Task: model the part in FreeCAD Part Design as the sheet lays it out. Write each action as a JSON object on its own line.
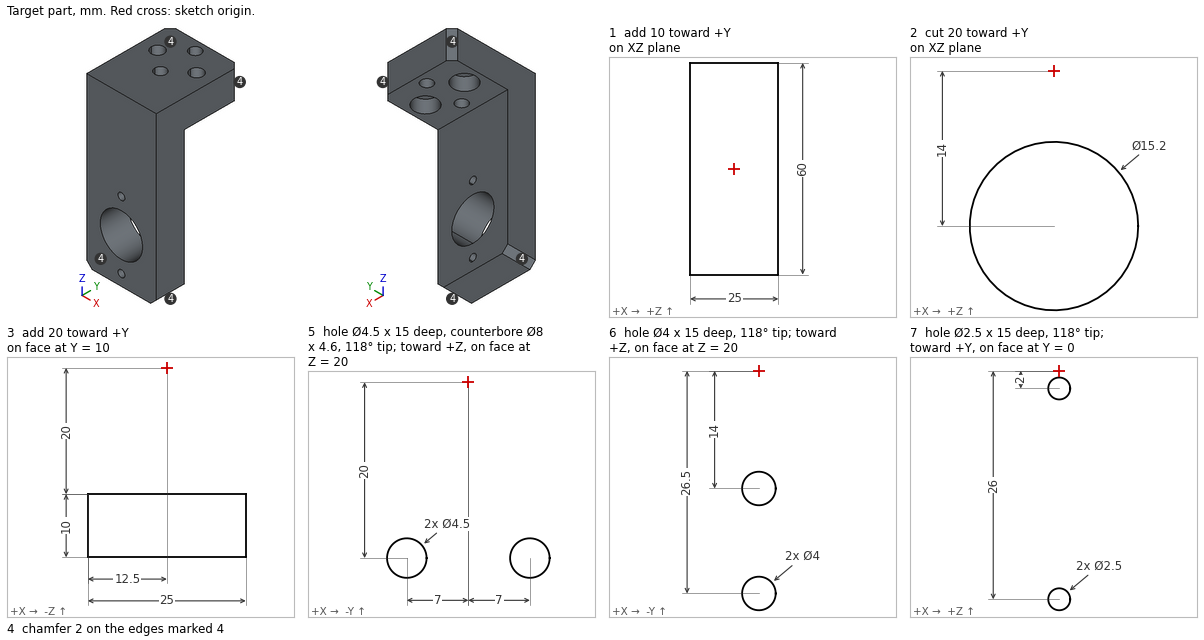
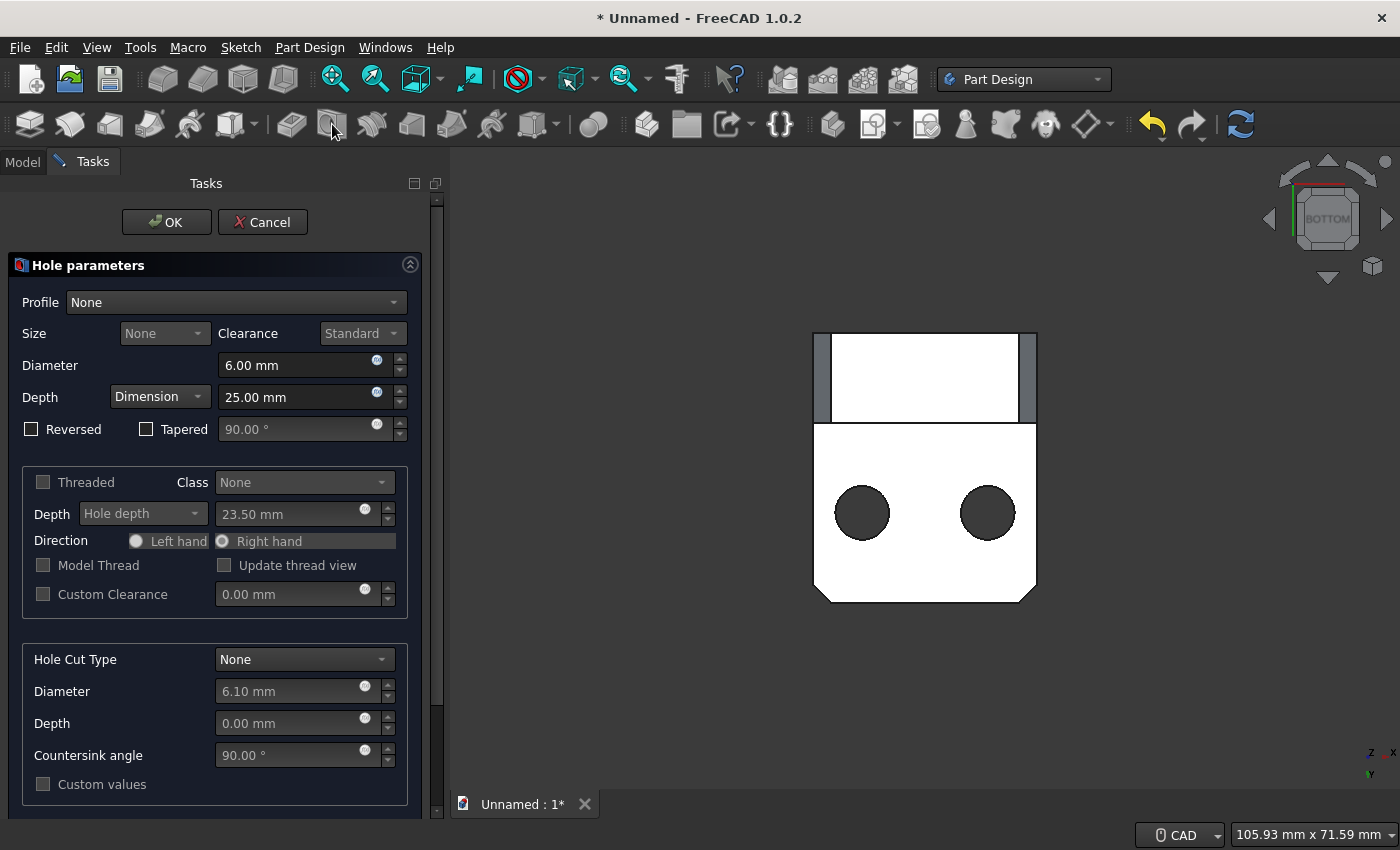
{"action": "triple_click", "coordinate": [305, 365]}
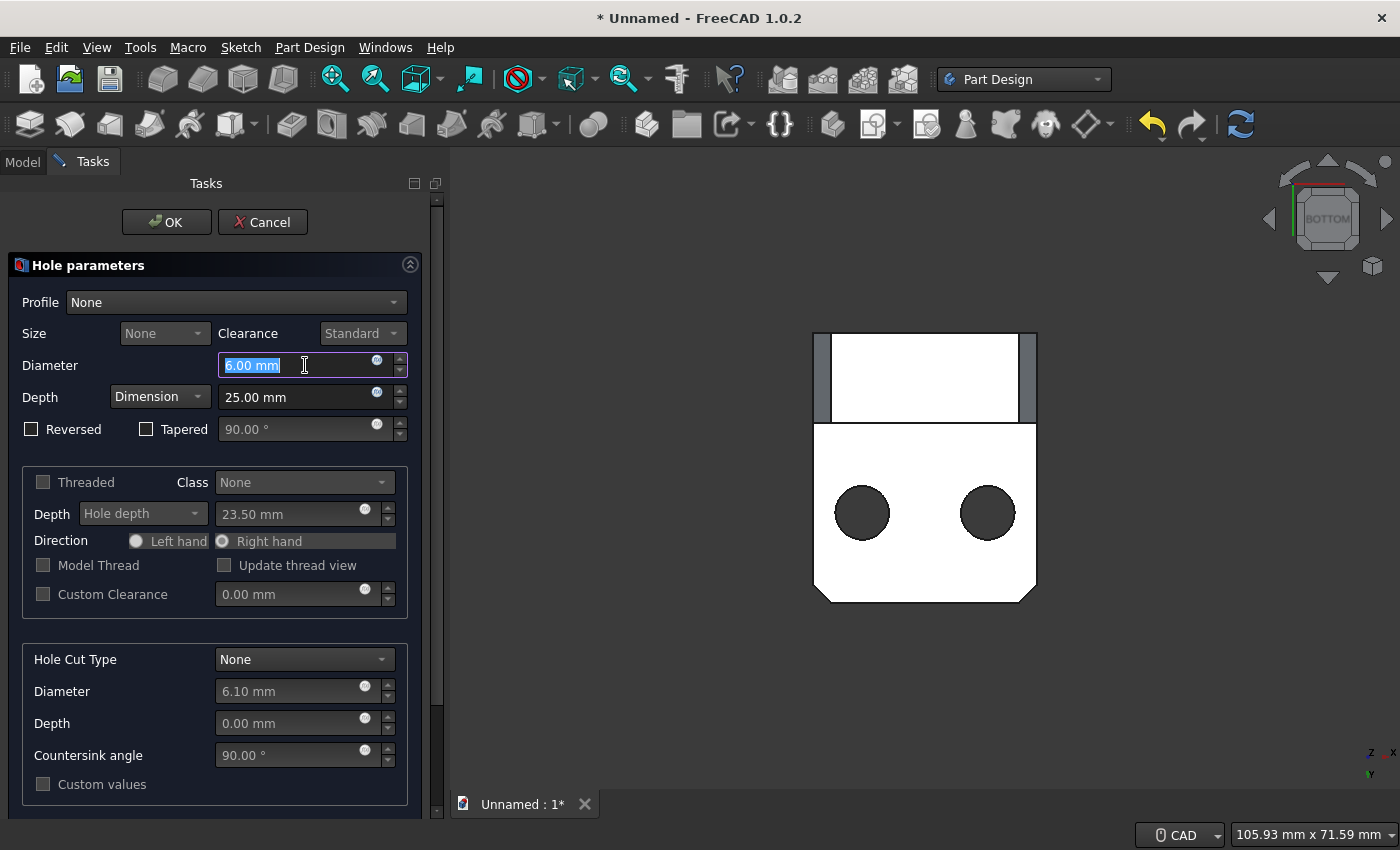
{"action": "type", "text": "4.5"}
{"action": "key", "text": "Tab"}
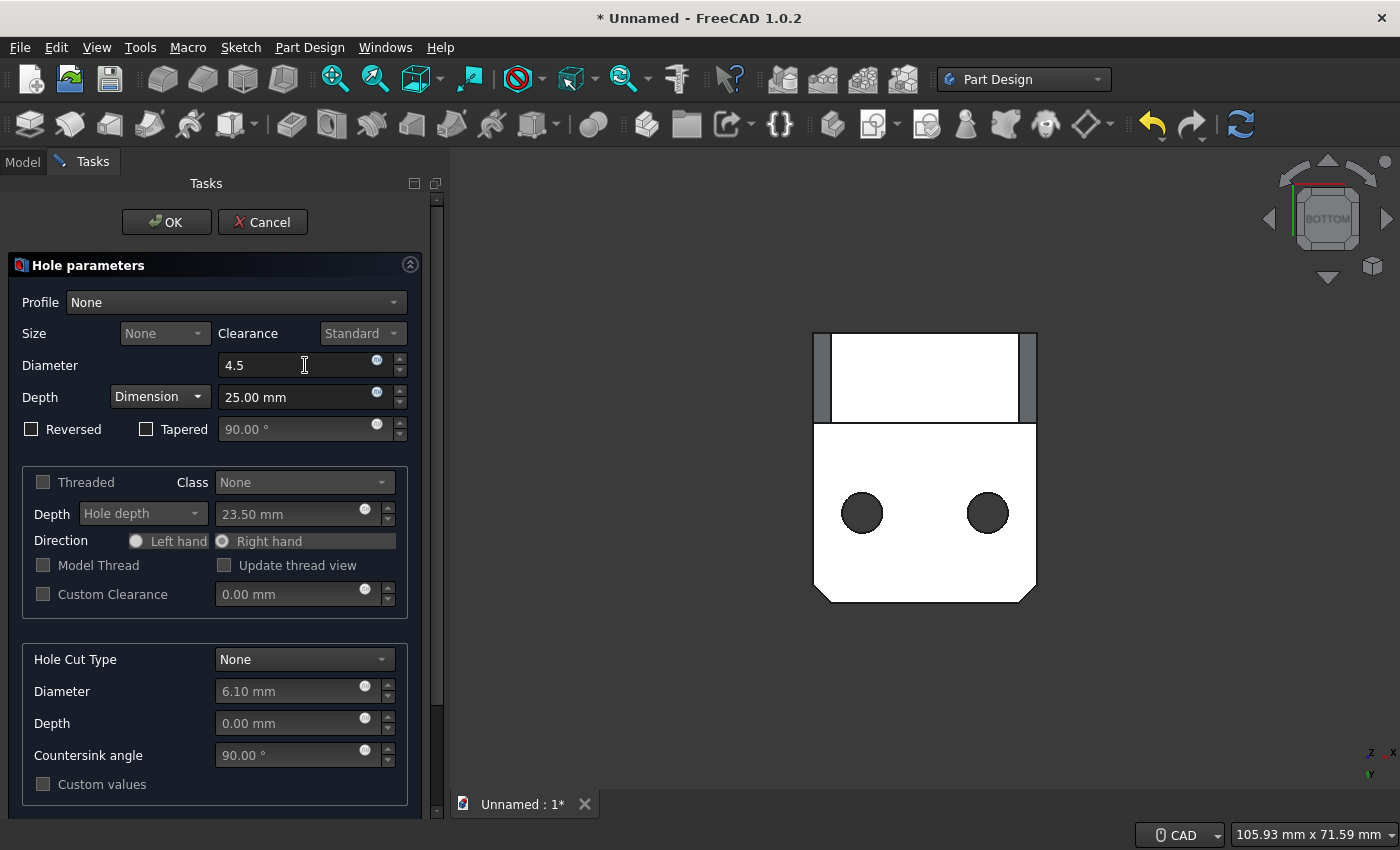
{"action": "triple_click", "coordinate": [305, 397]}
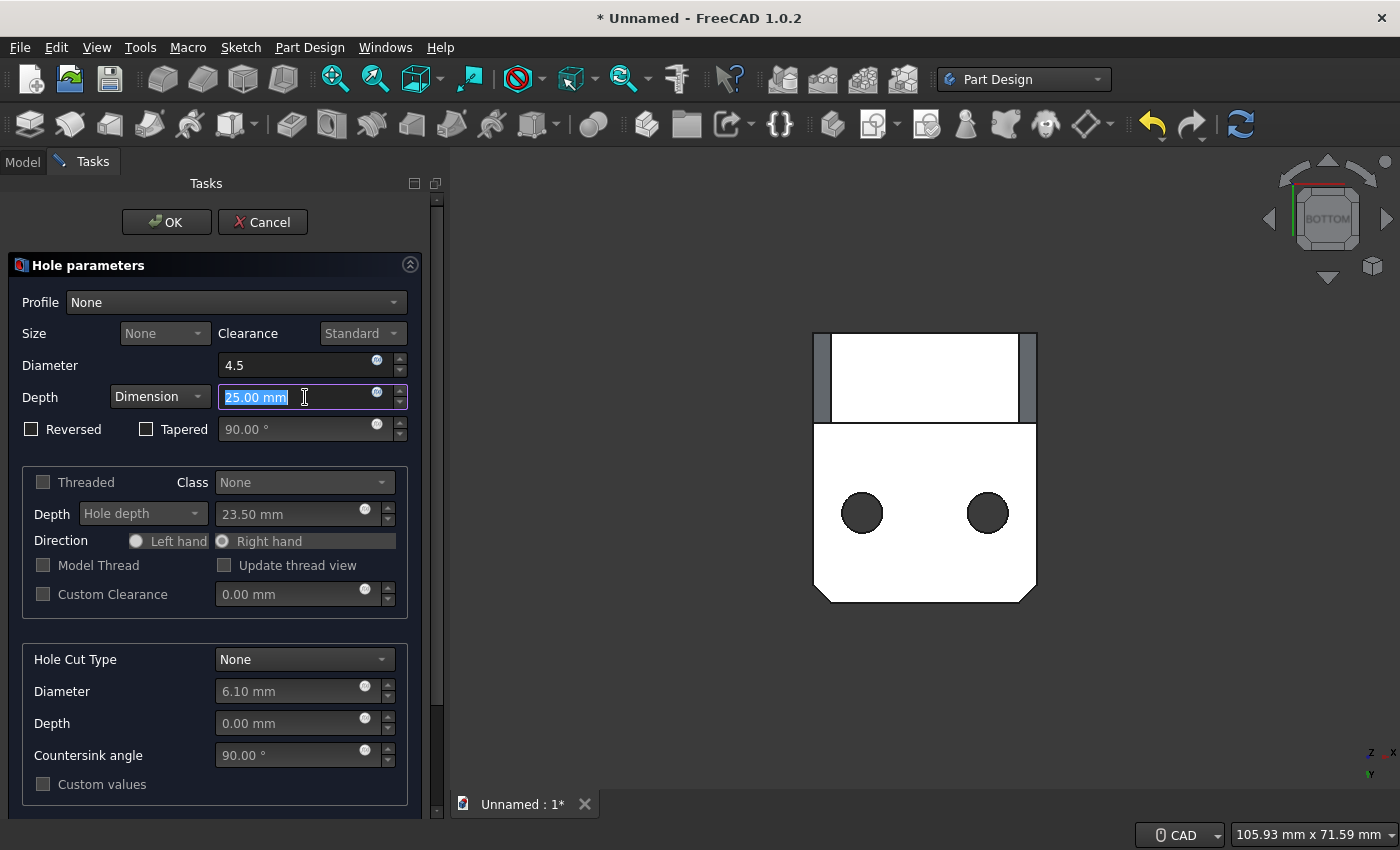
{"action": "type", "text": "15"}
{"action": "key", "text": "Tab"}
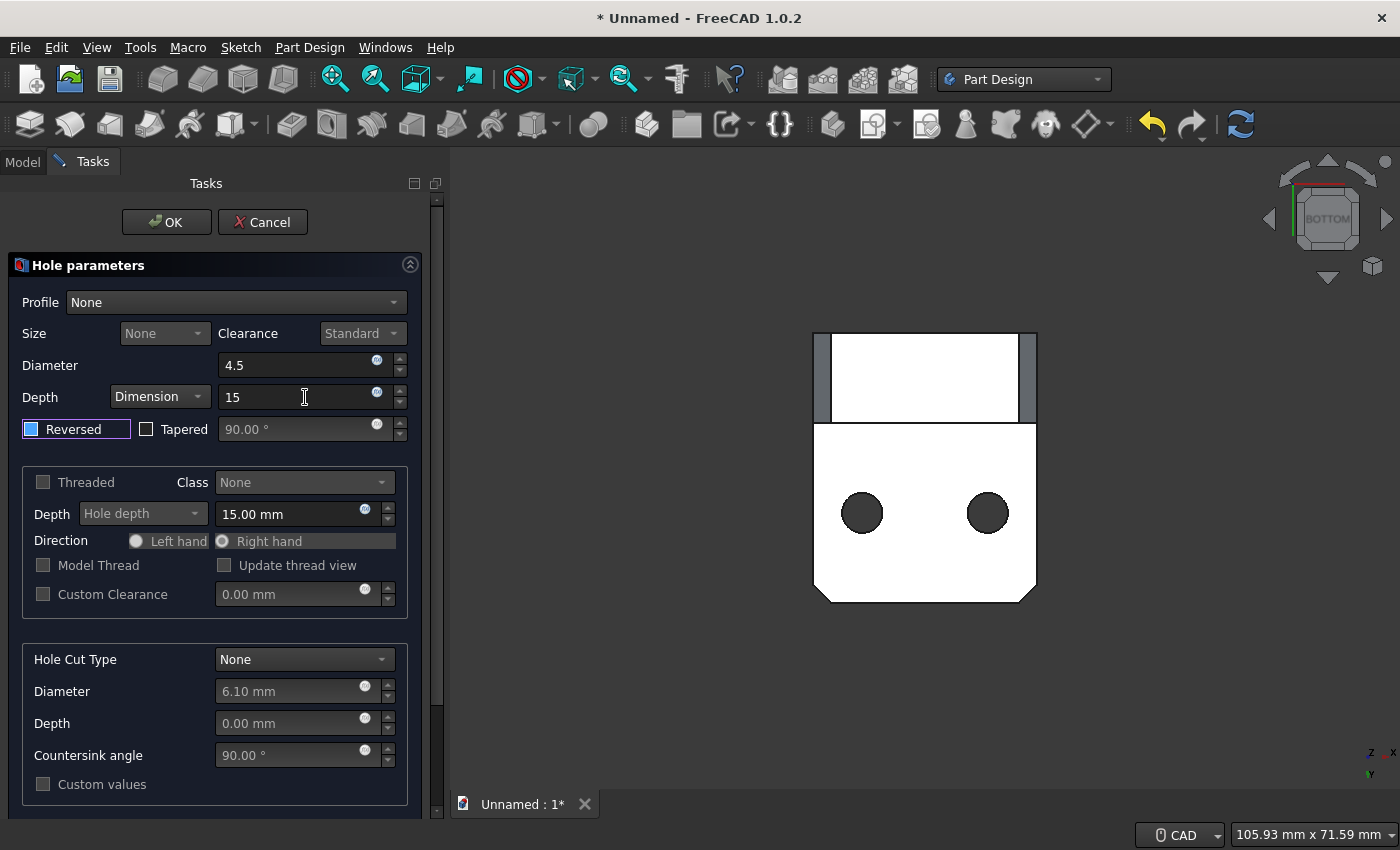
{"action": "left_click", "coordinate": [306, 660]}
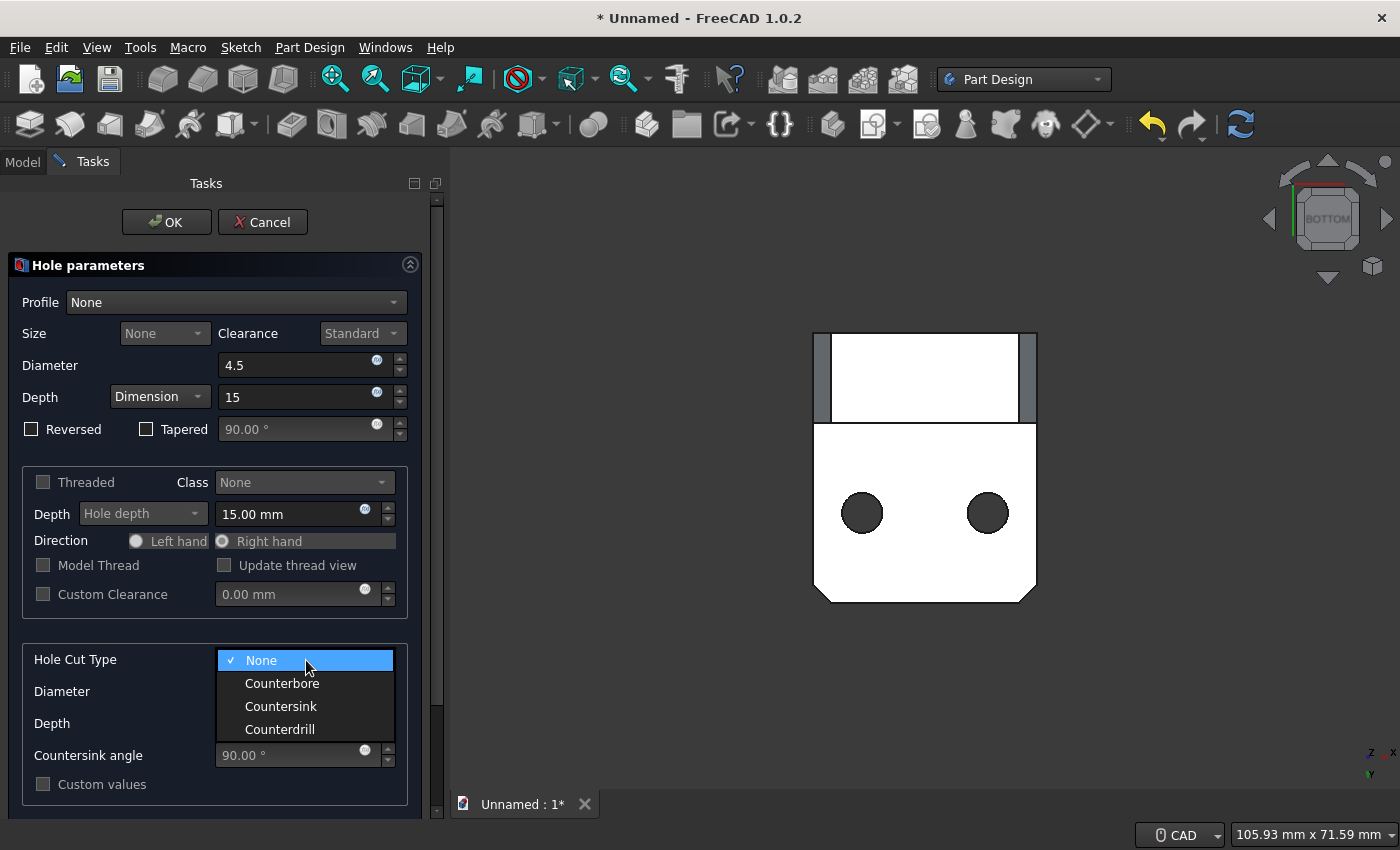
{"action": "left_click", "coordinate": [304, 684]}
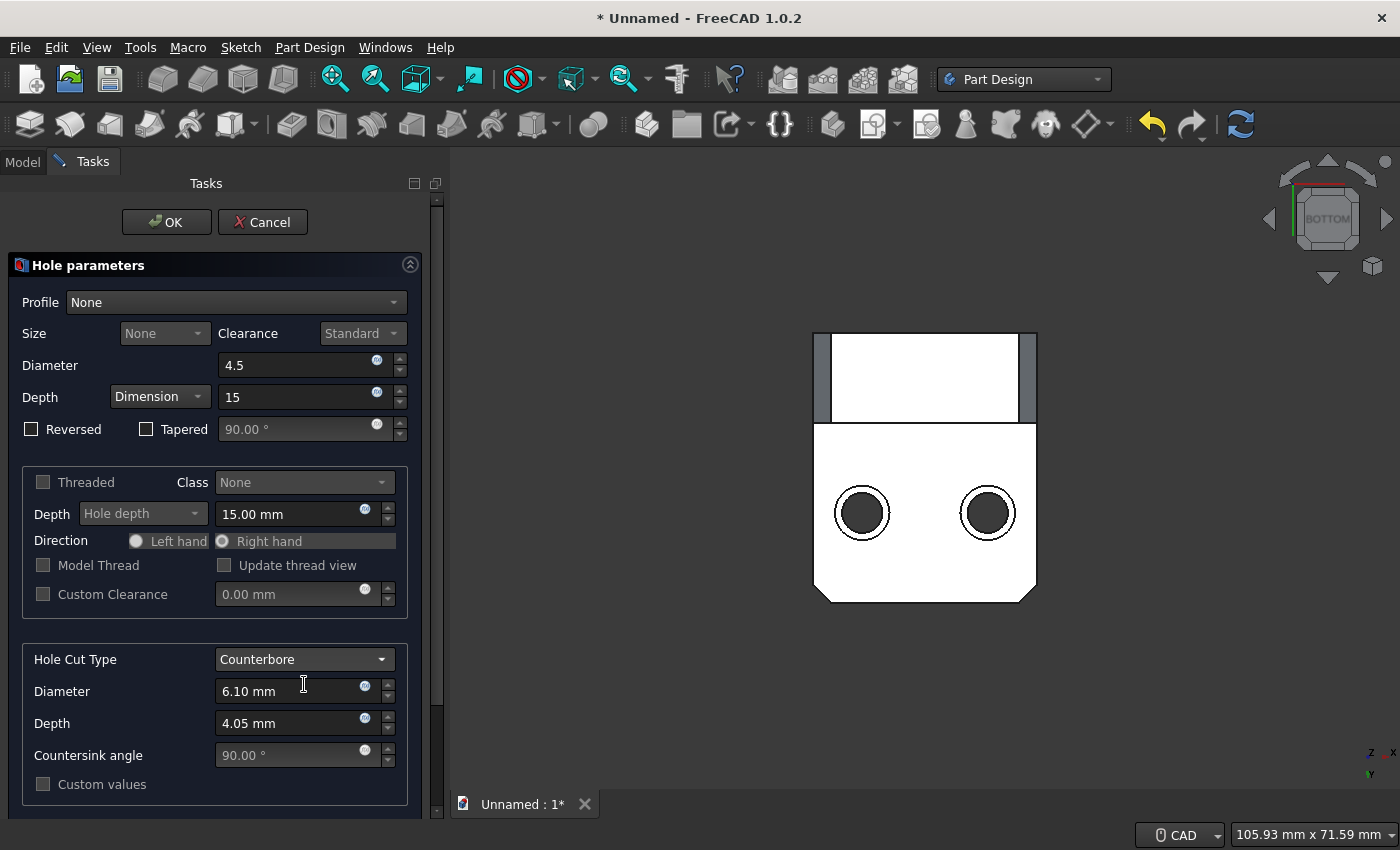
{"action": "triple_click", "coordinate": [298, 691]}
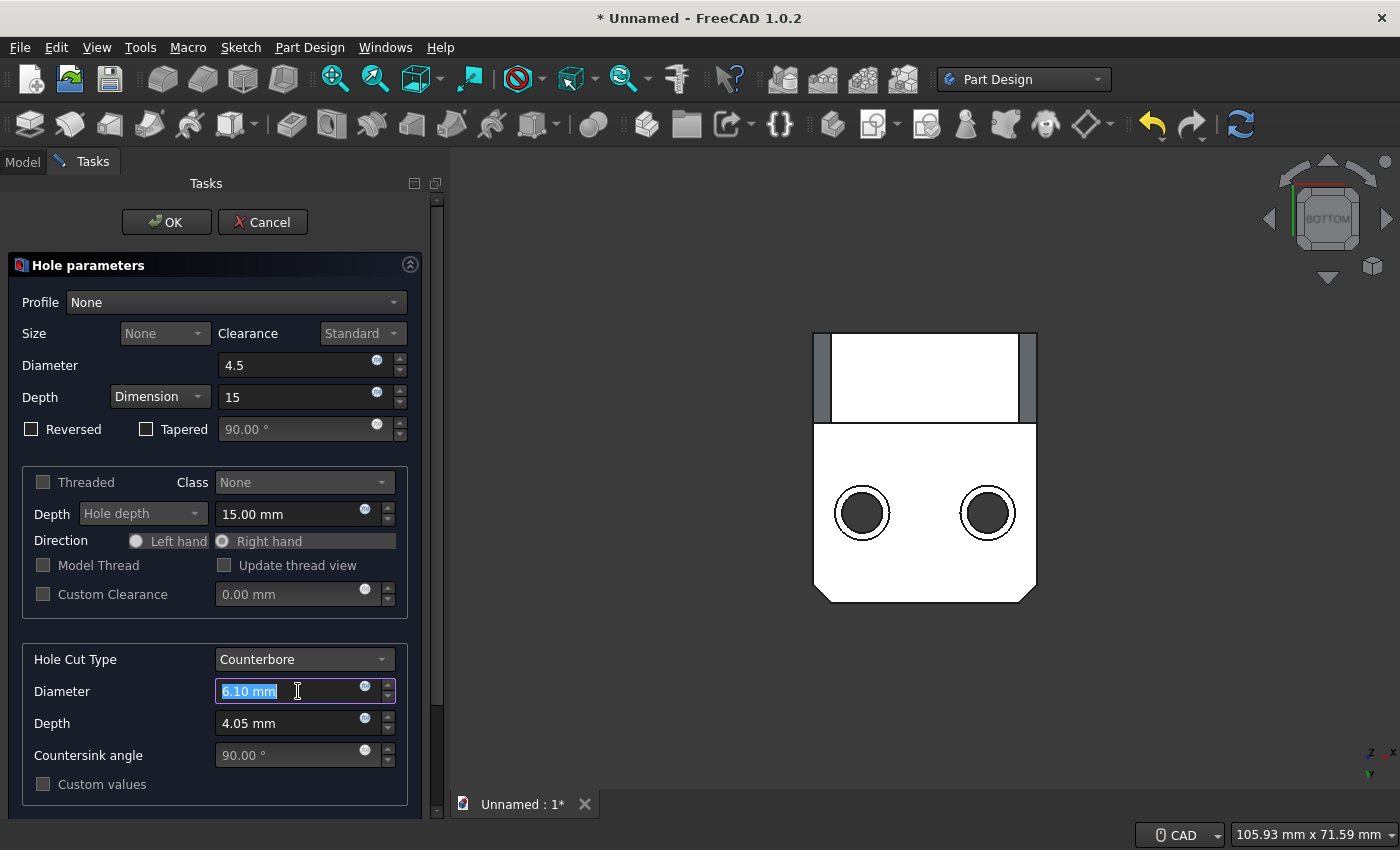
{"action": "type", "text": "8"}
{"action": "key", "text": "Tab"}